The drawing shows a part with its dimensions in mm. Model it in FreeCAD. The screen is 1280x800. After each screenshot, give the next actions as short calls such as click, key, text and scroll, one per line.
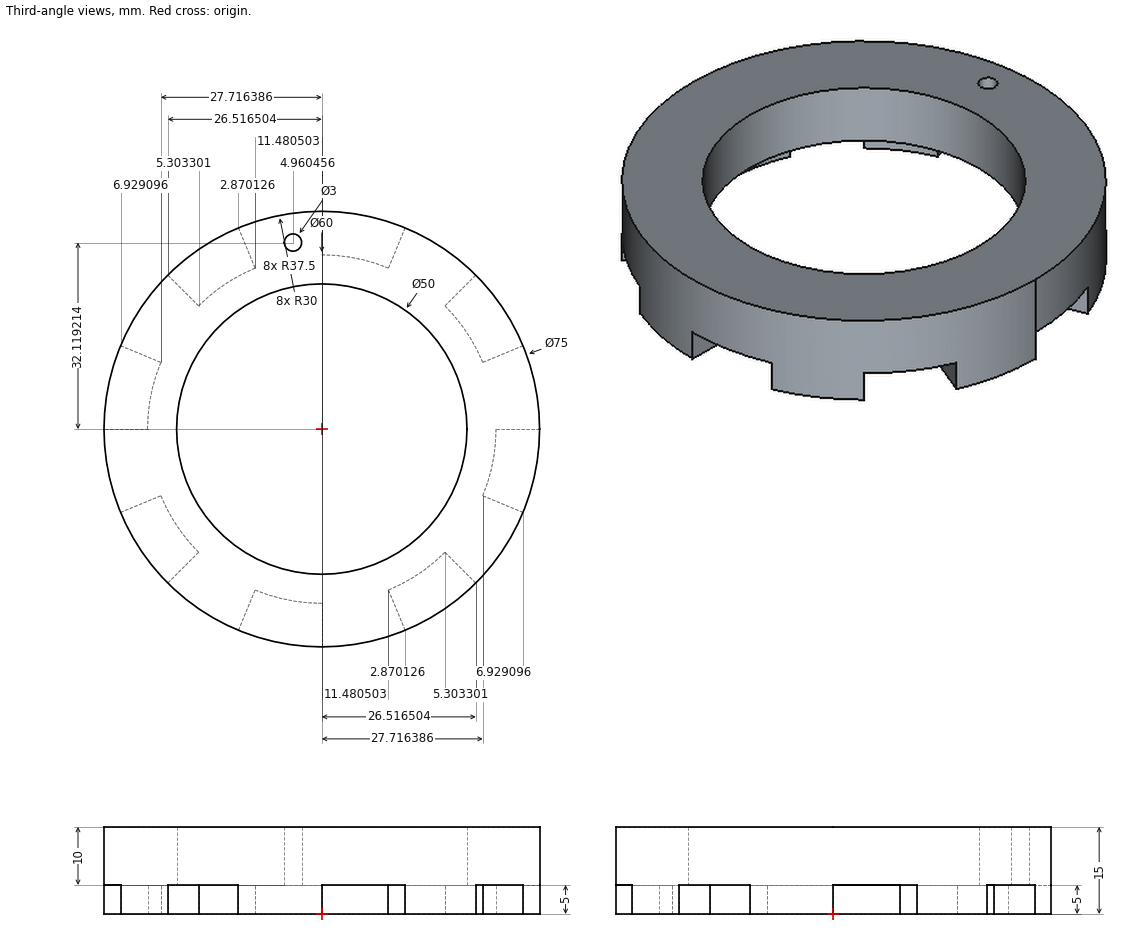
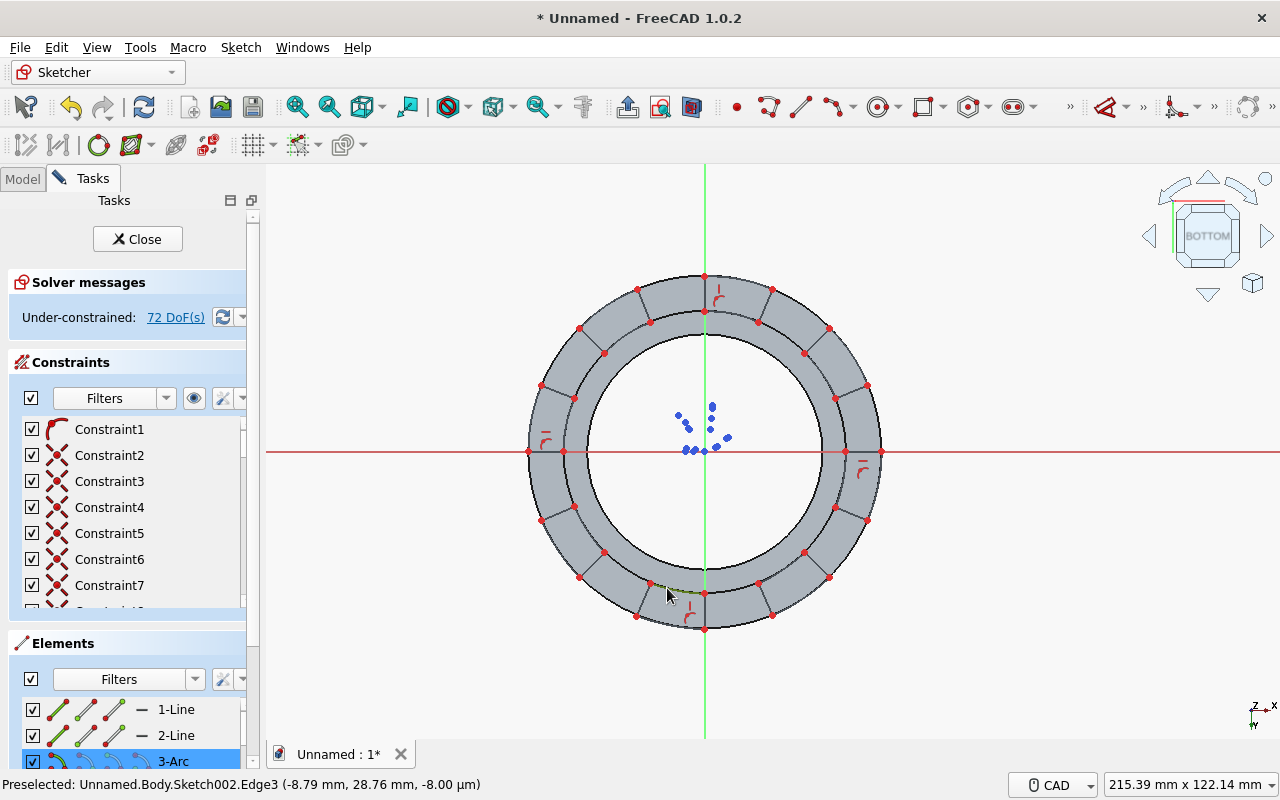
click(657, 622)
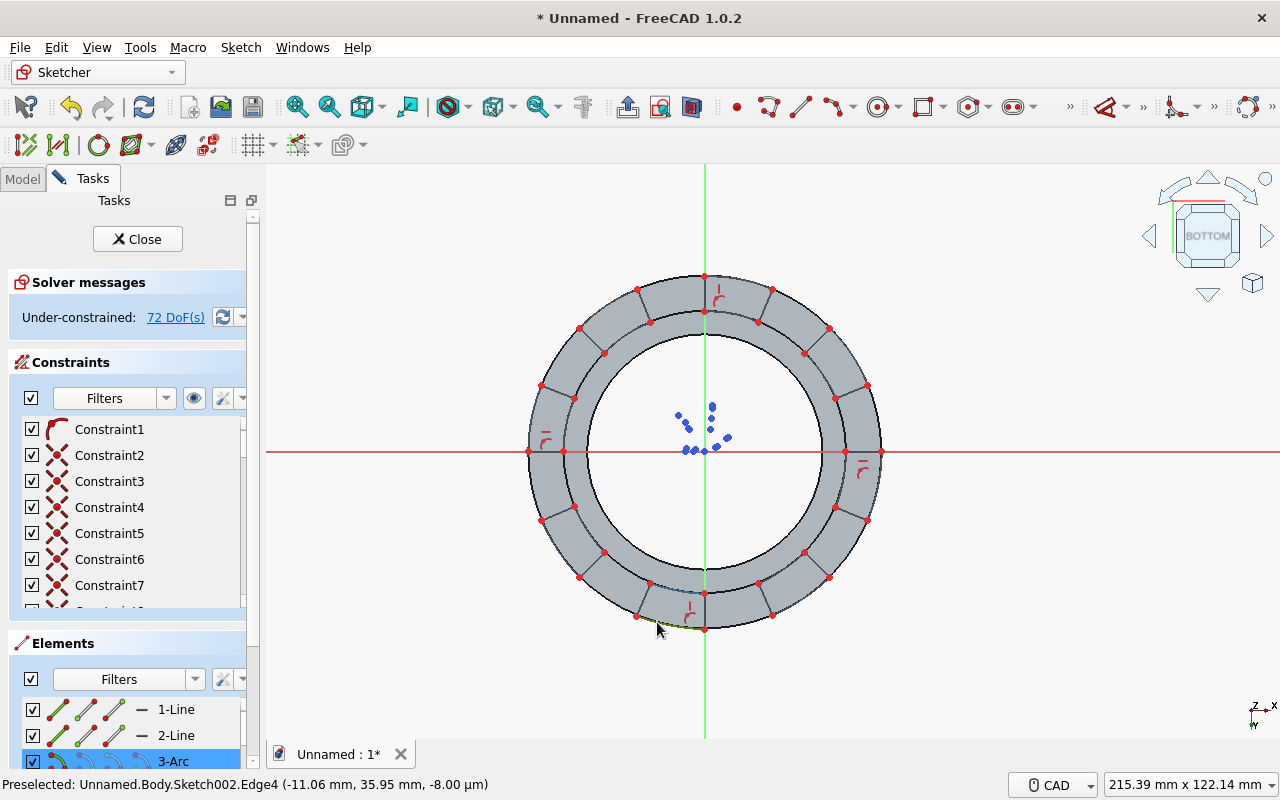
key(c)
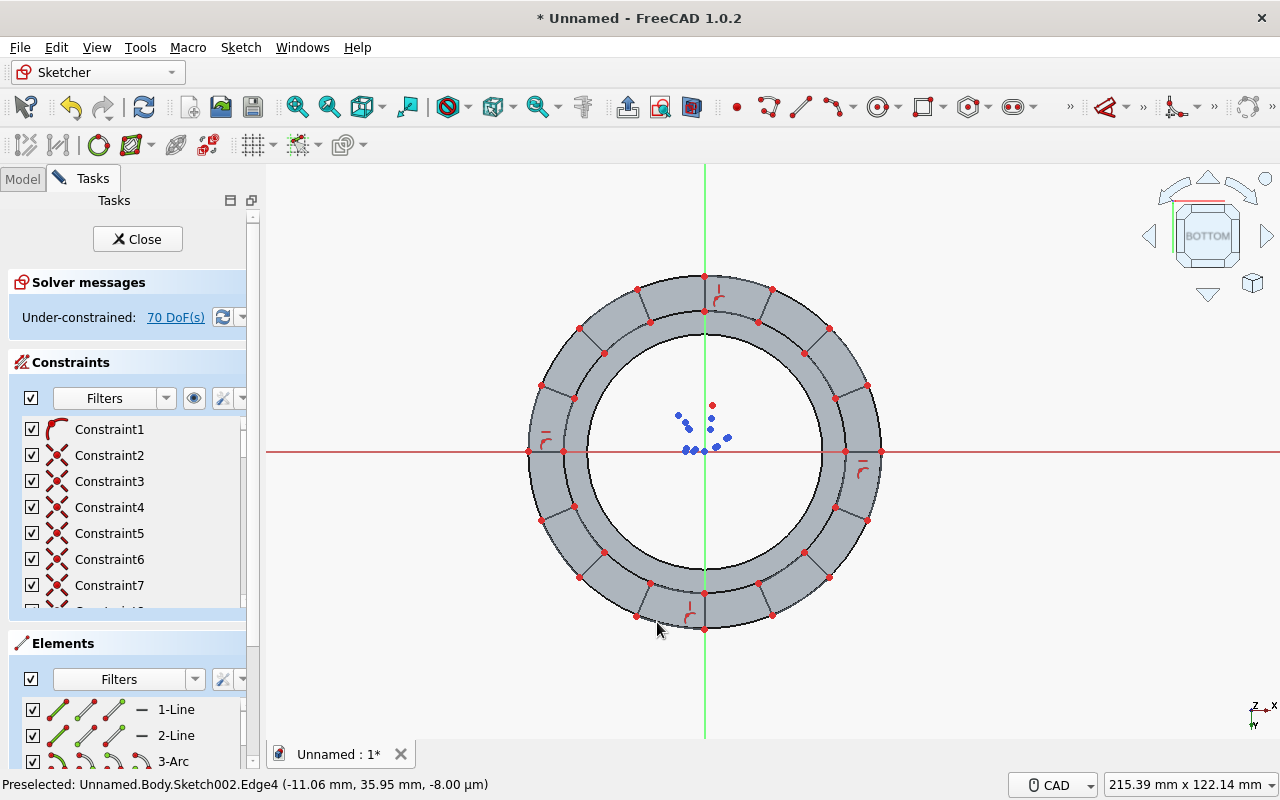
click(667, 588)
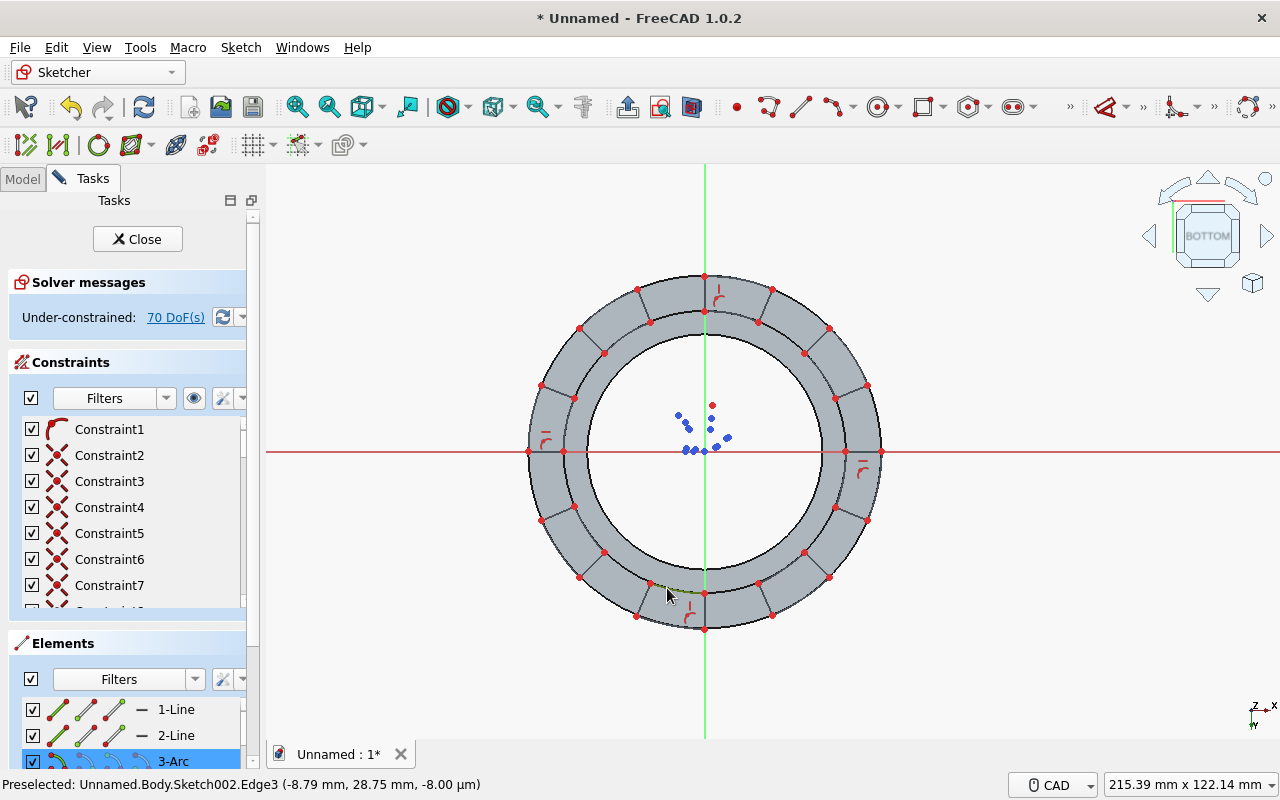
click(582, 522)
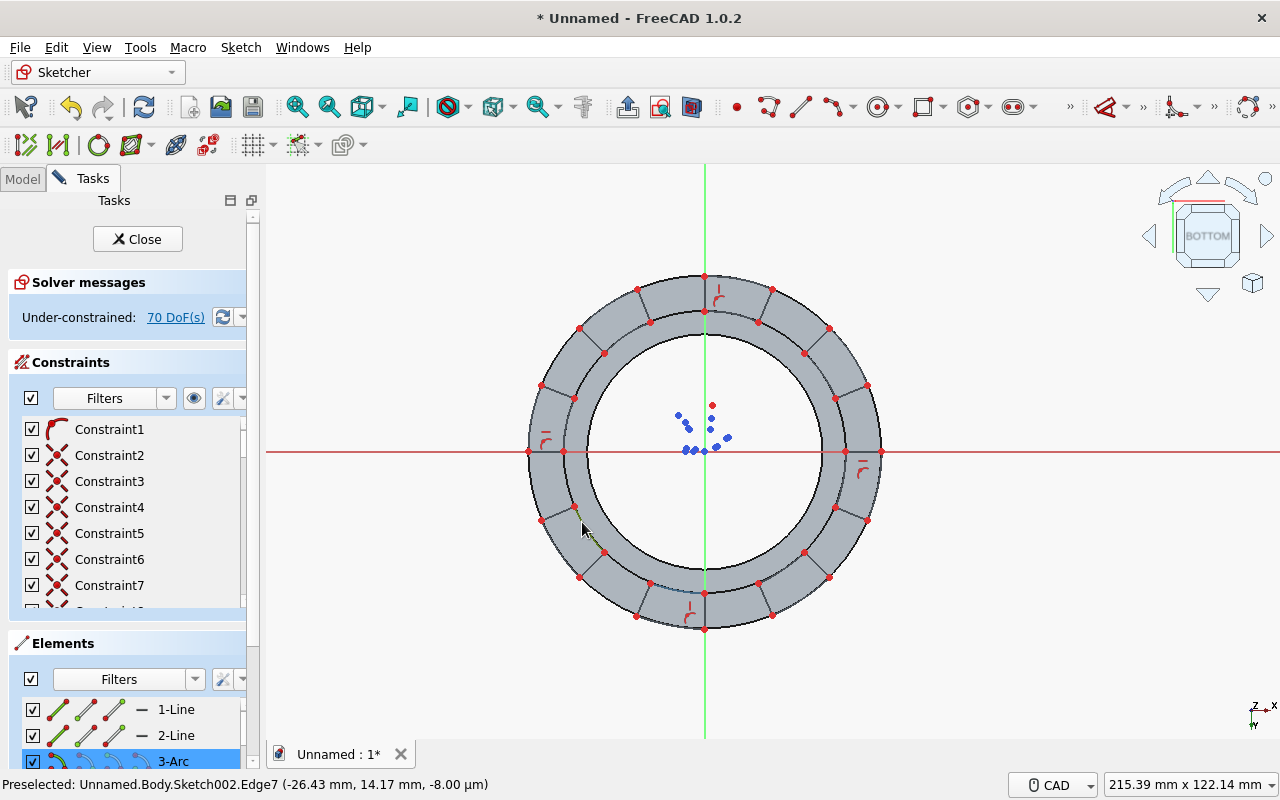
key(c)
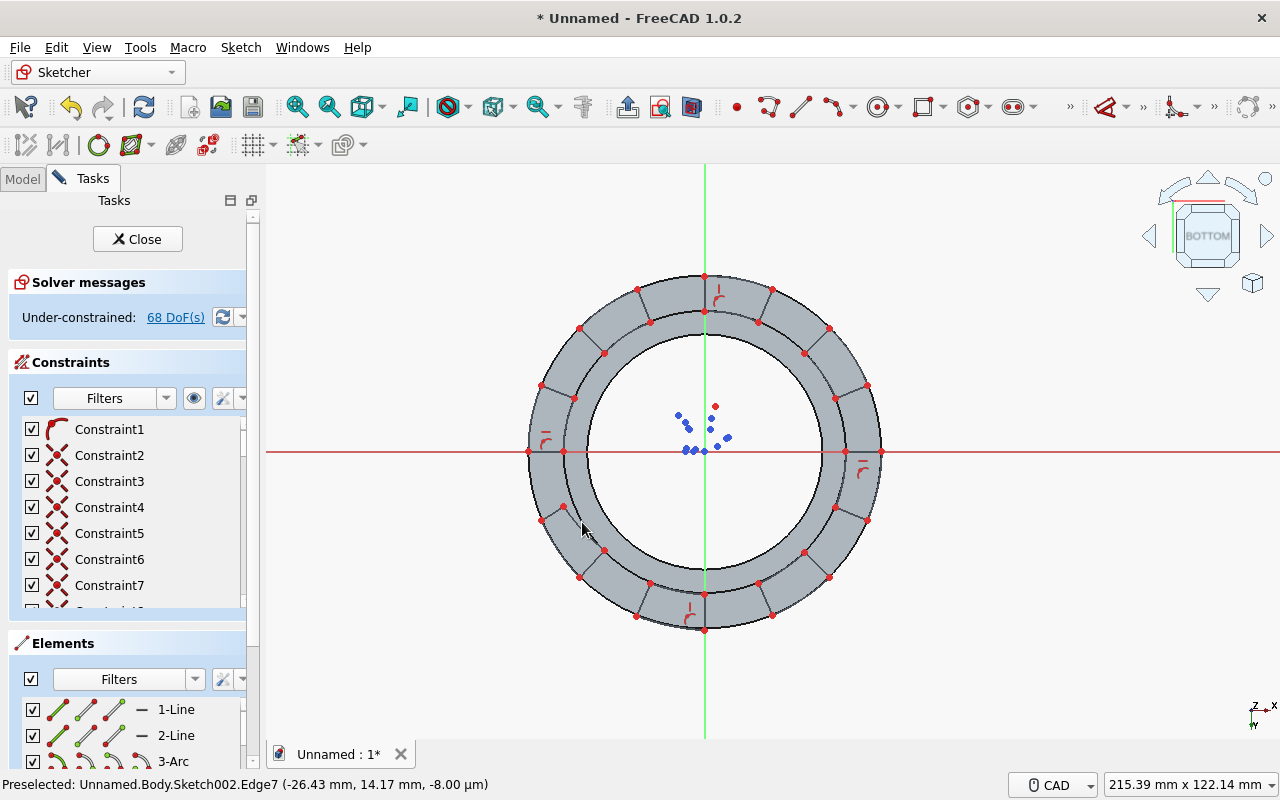
click(667, 588)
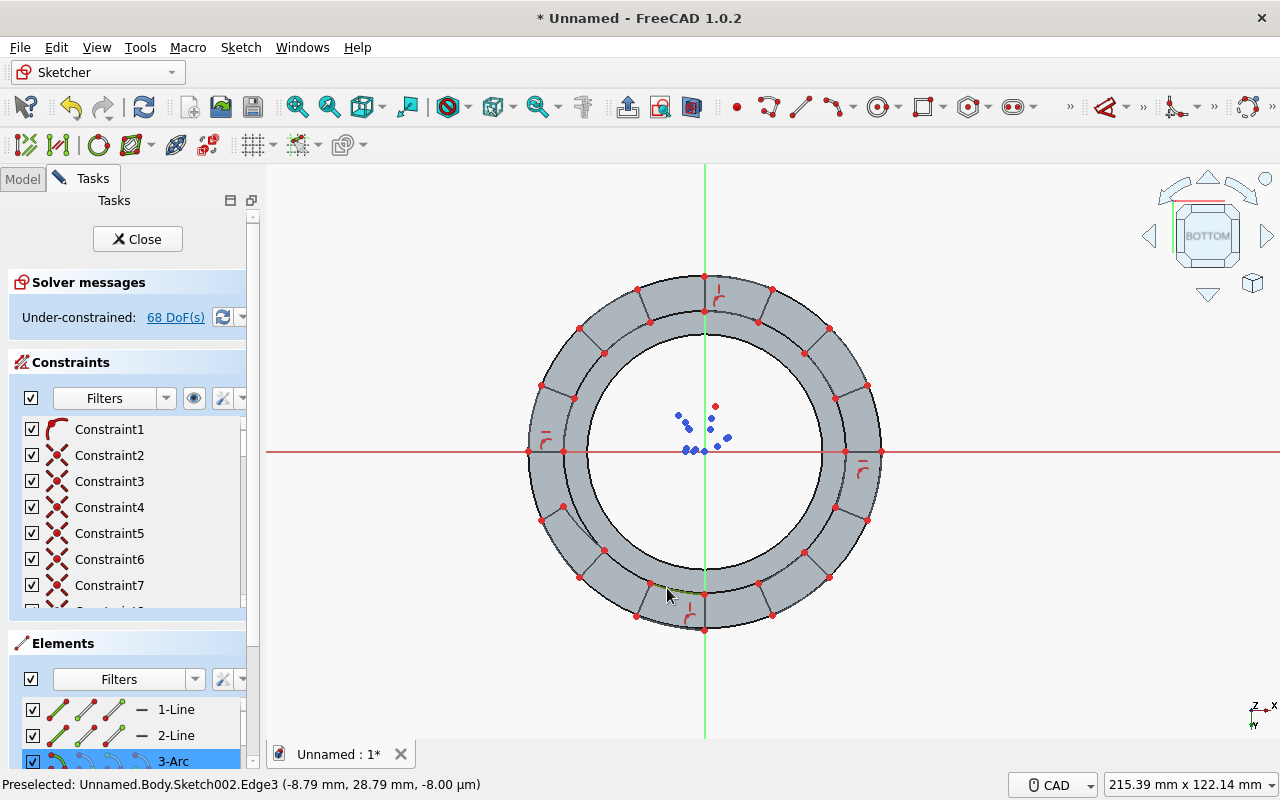
click(551, 539)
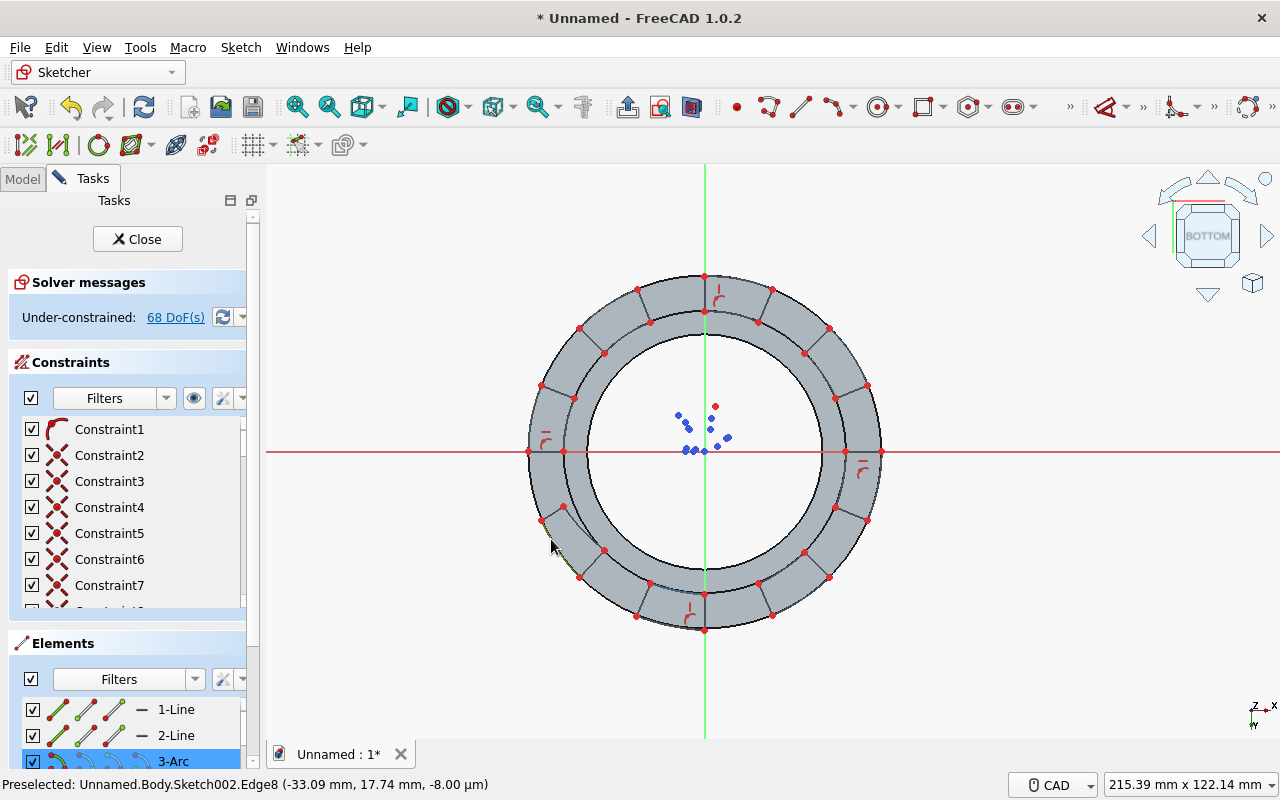
key(c)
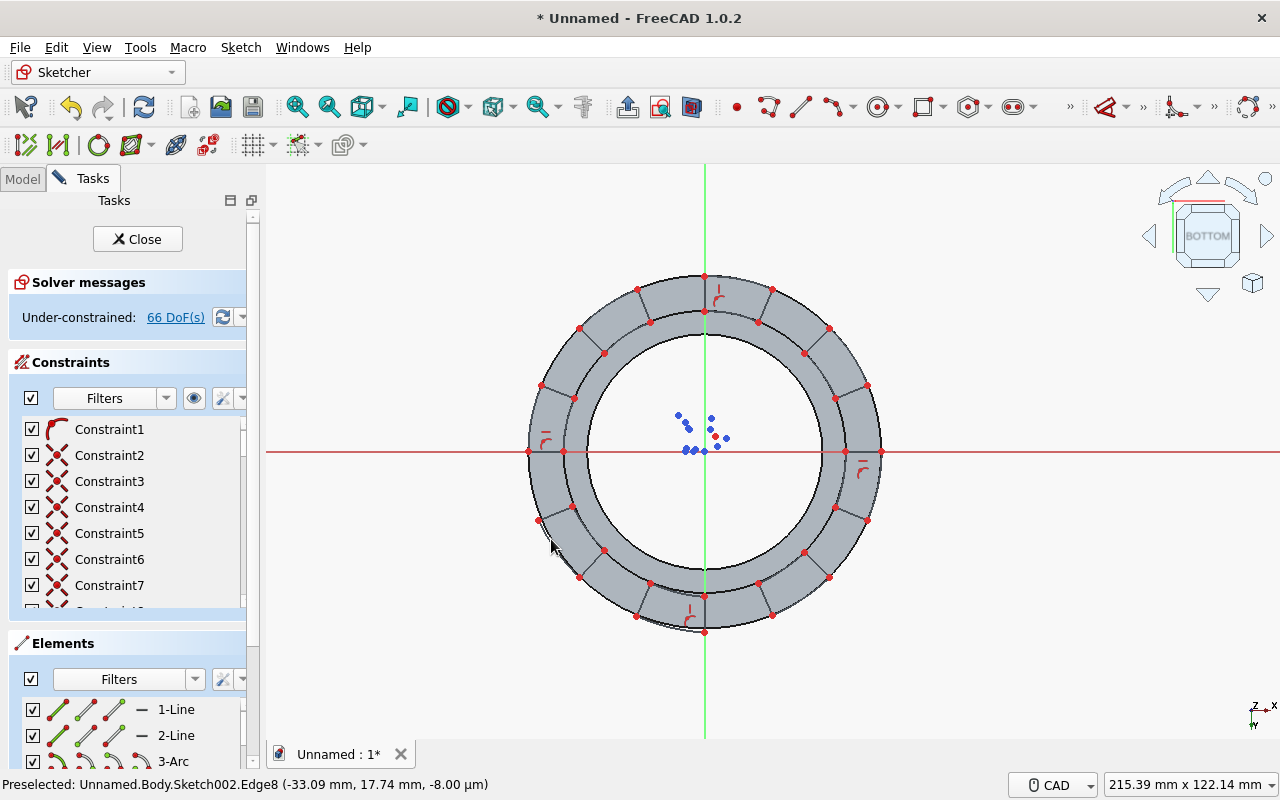
click(666, 589)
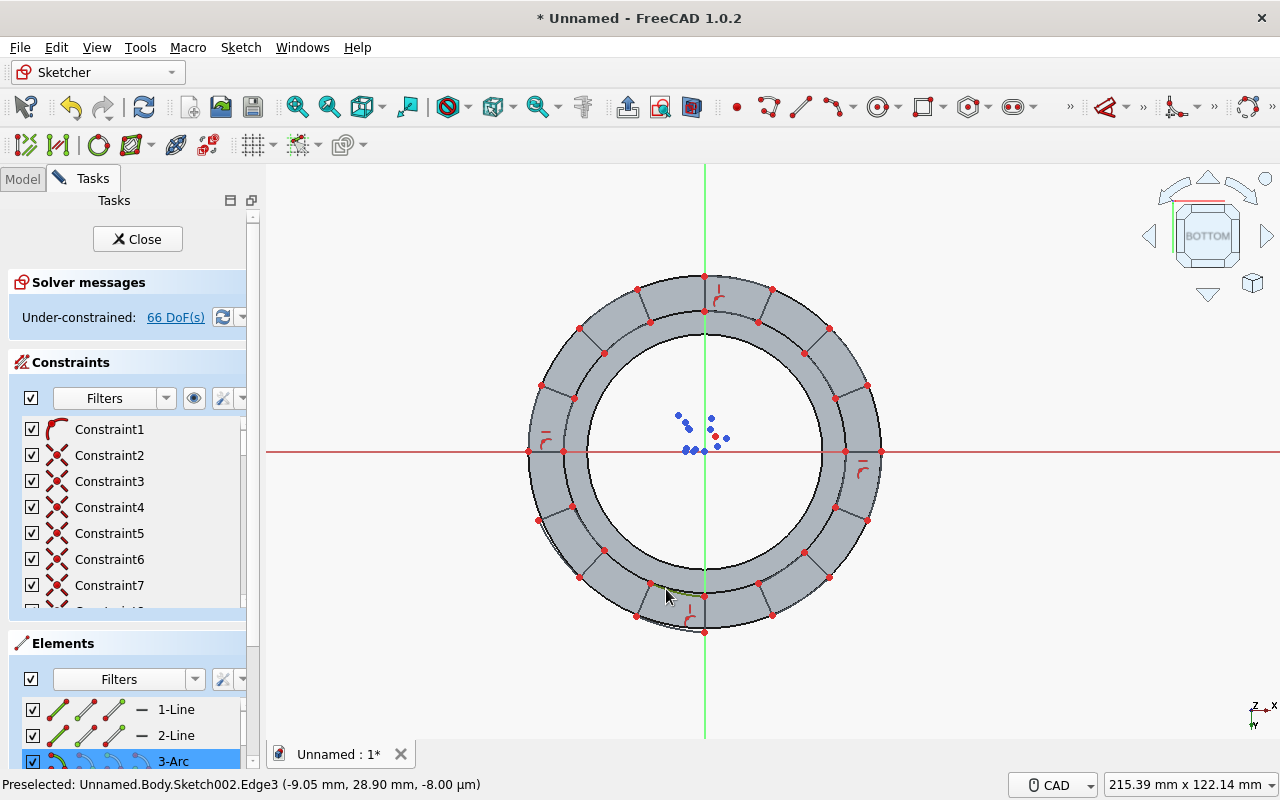
click(569, 414)